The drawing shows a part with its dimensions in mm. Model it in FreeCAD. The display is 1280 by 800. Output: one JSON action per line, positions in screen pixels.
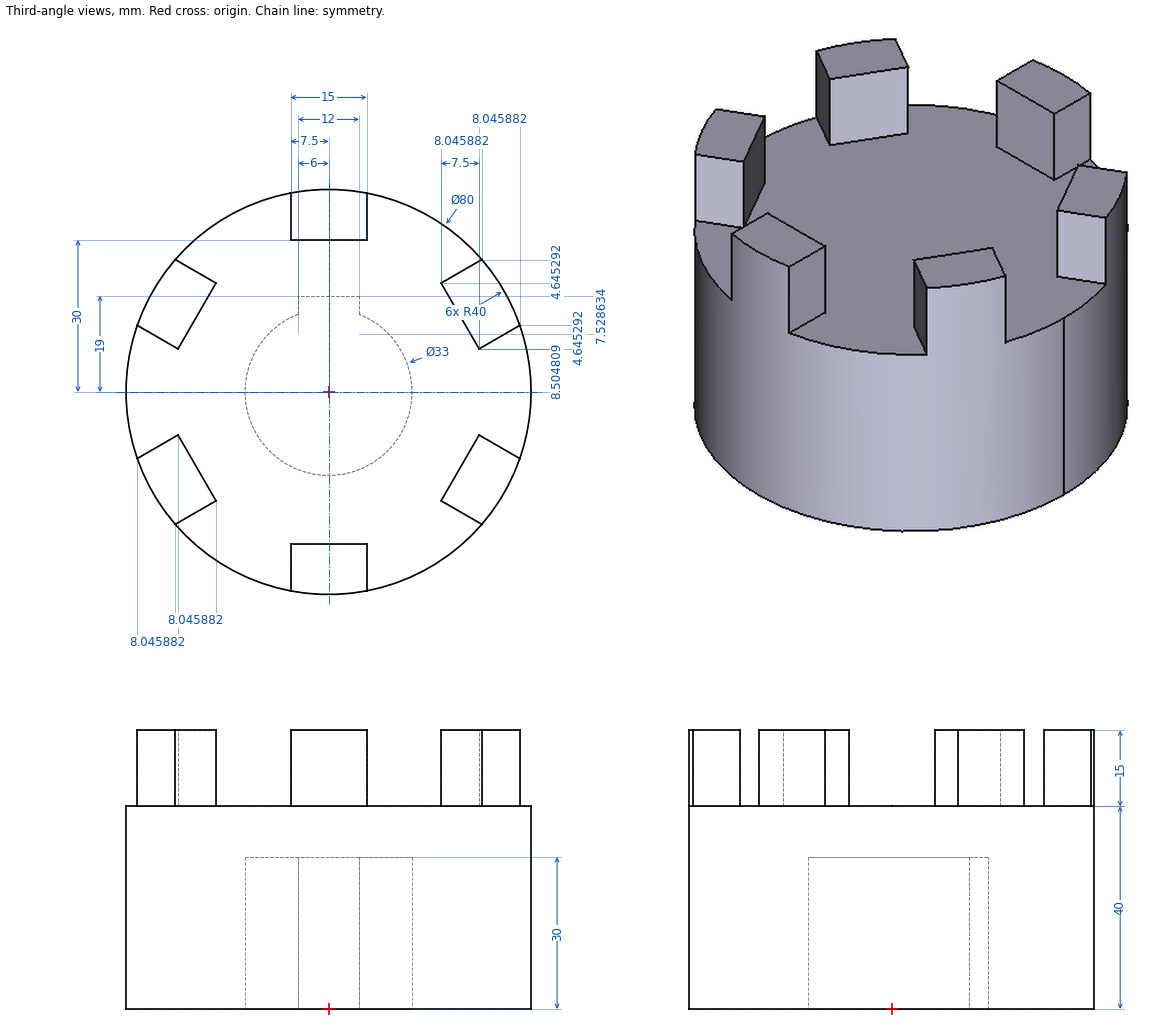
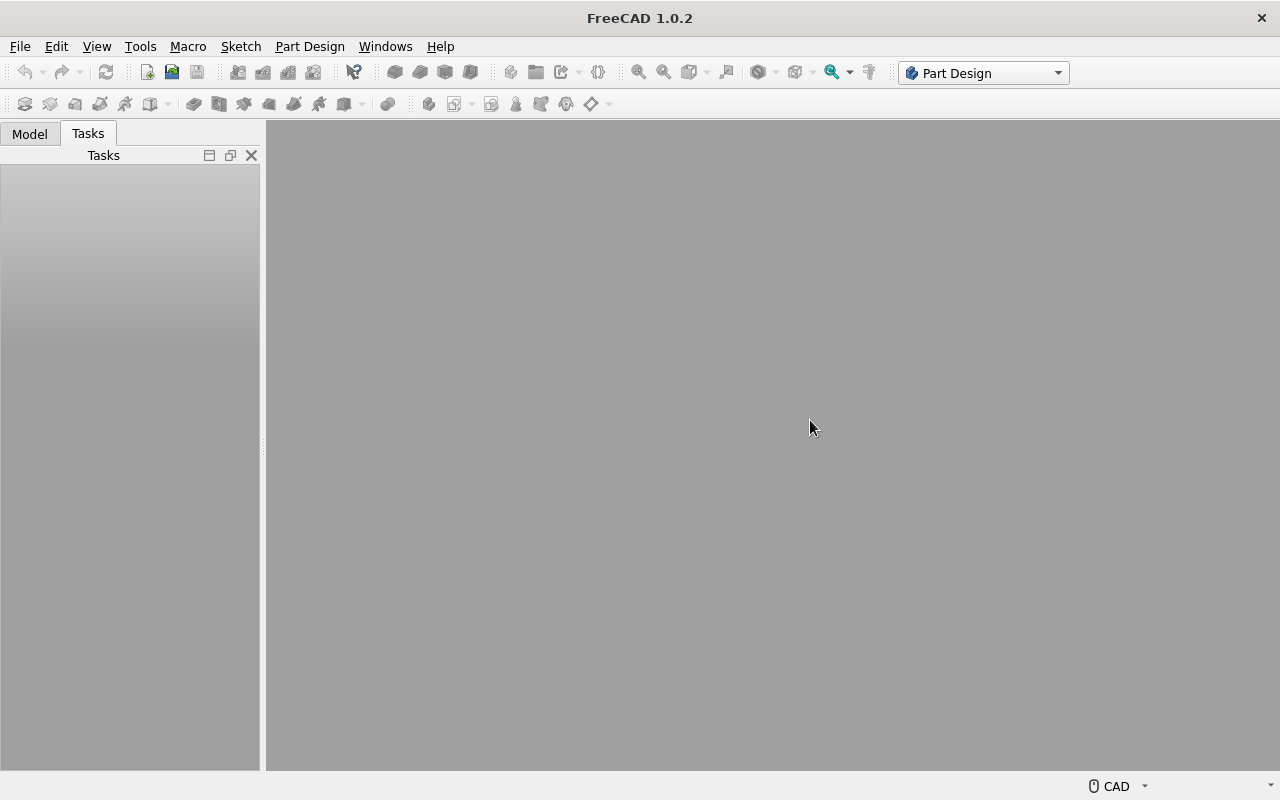
{"action": "key", "text": "ctrl+n"}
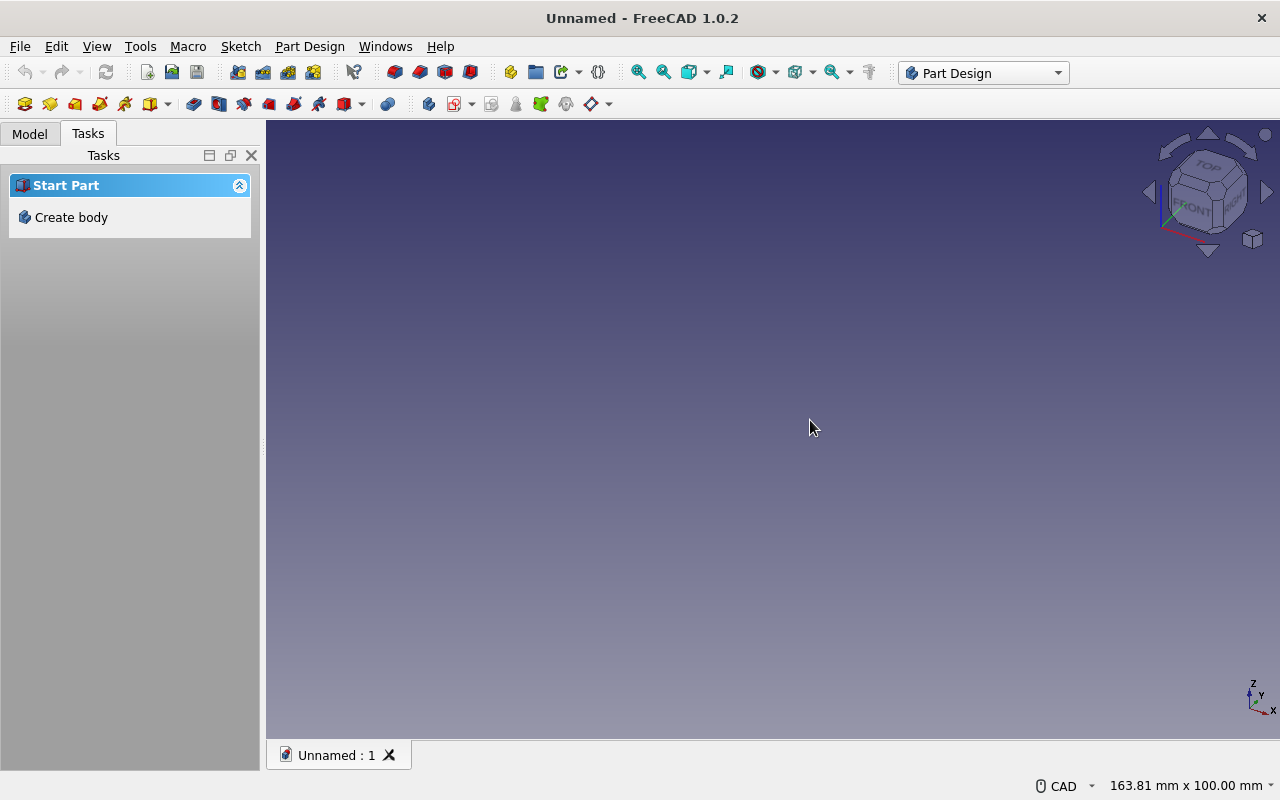
{"action": "left_click", "coordinate": [454, 104]}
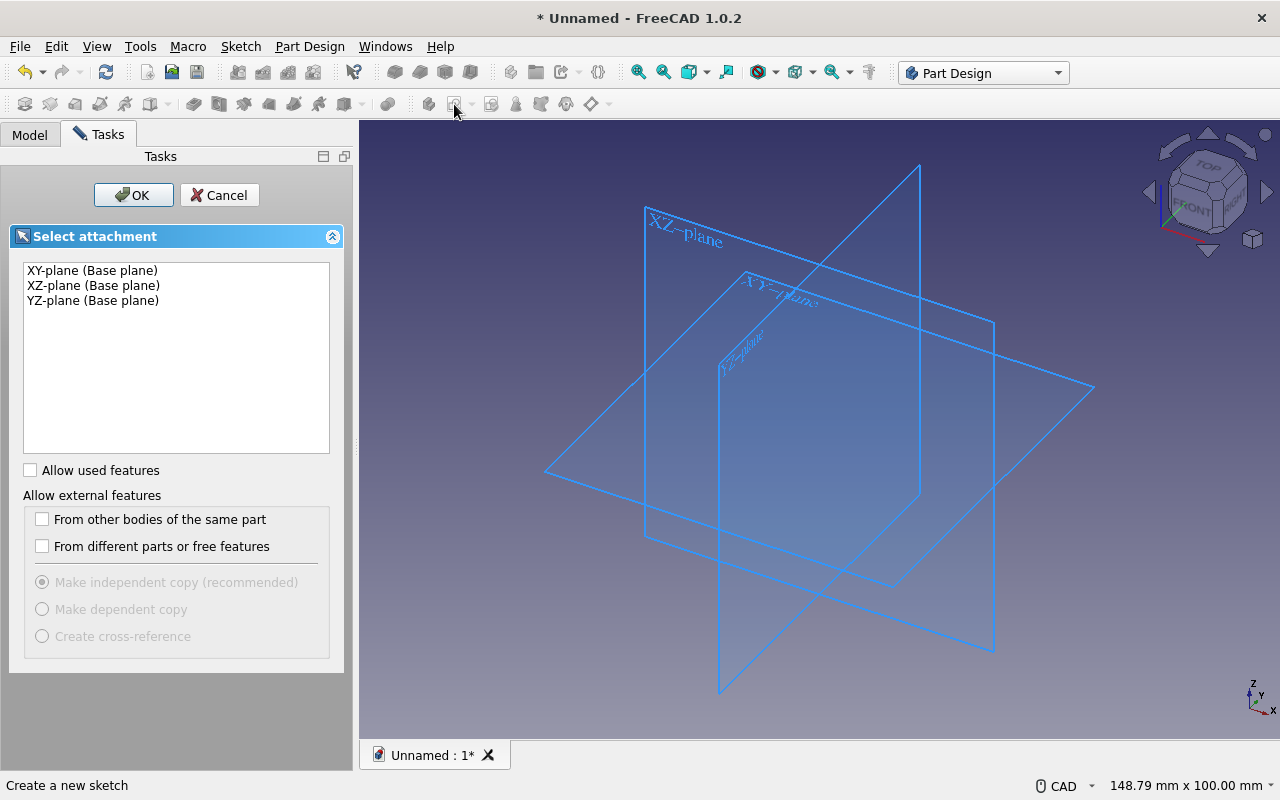
{"action": "left_click", "coordinate": [84, 270]}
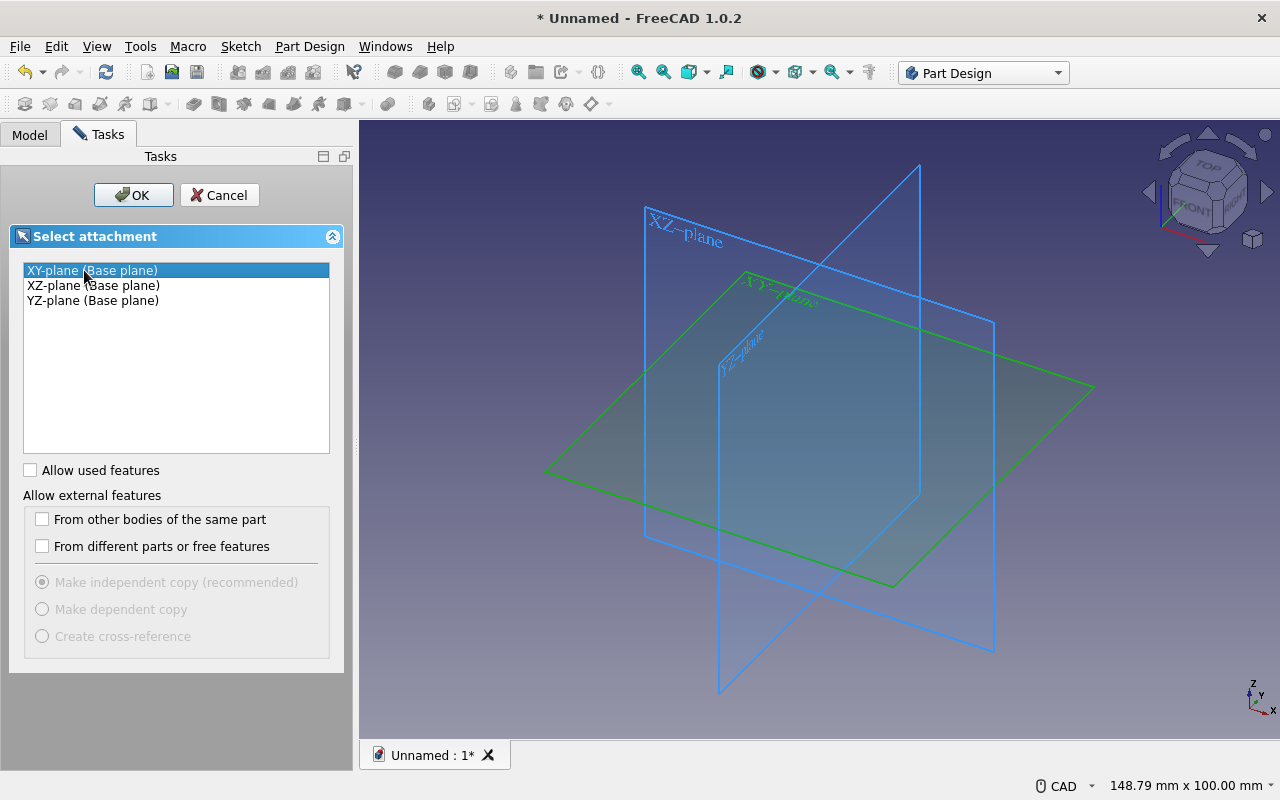
{"action": "left_click", "coordinate": [134, 195]}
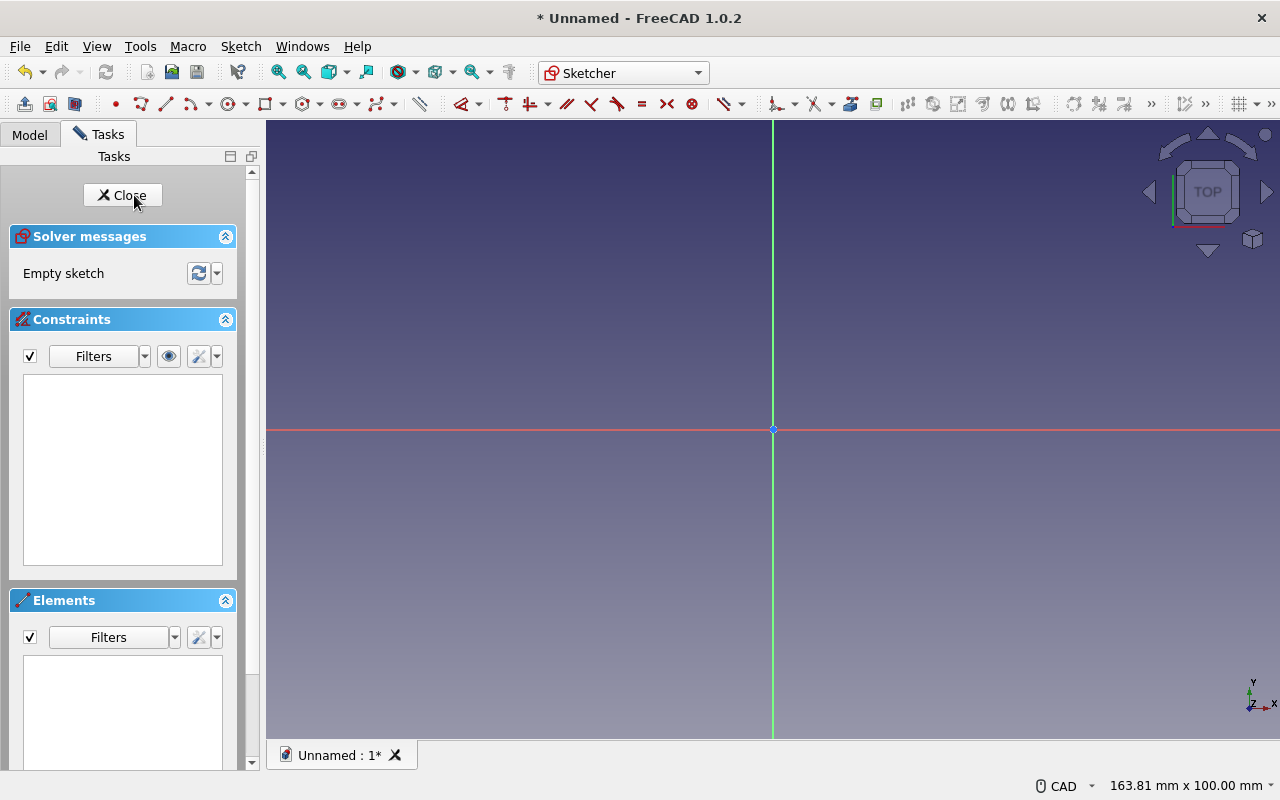
{"action": "key", "text": "g c"}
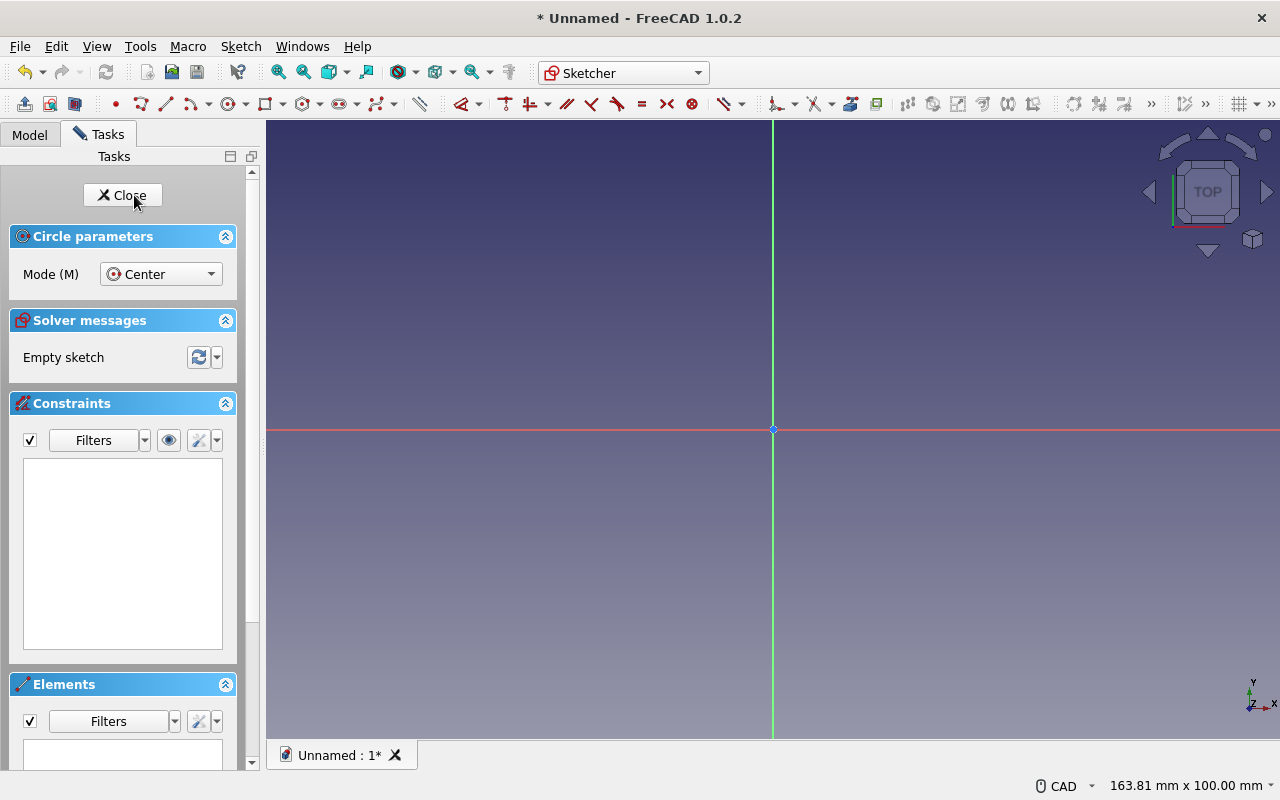
{"action": "left_click", "coordinate": [773, 430]}
{"action": "mouse_move", "coordinate": [948, 254]}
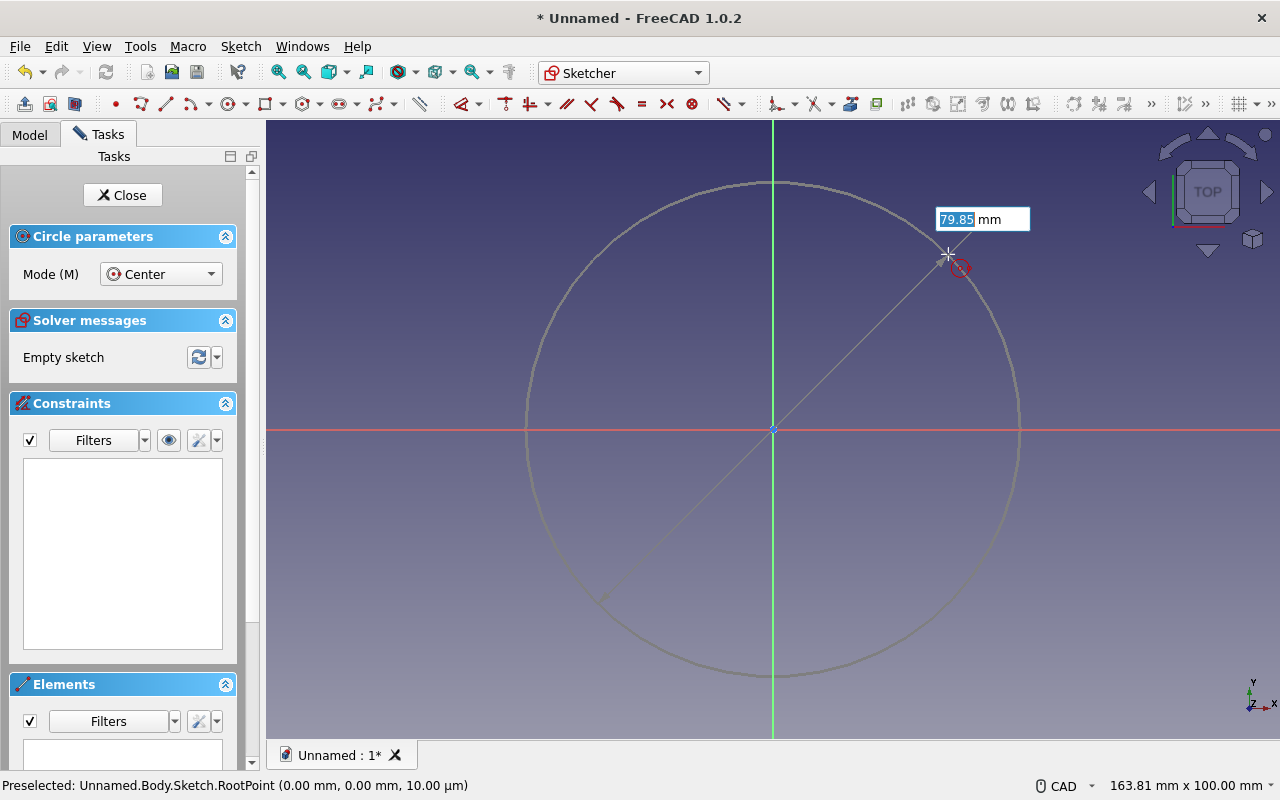
{"action": "type", "text": "80"}
{"action": "key", "text": "Return"}
{"action": "key", "text": "Escape"}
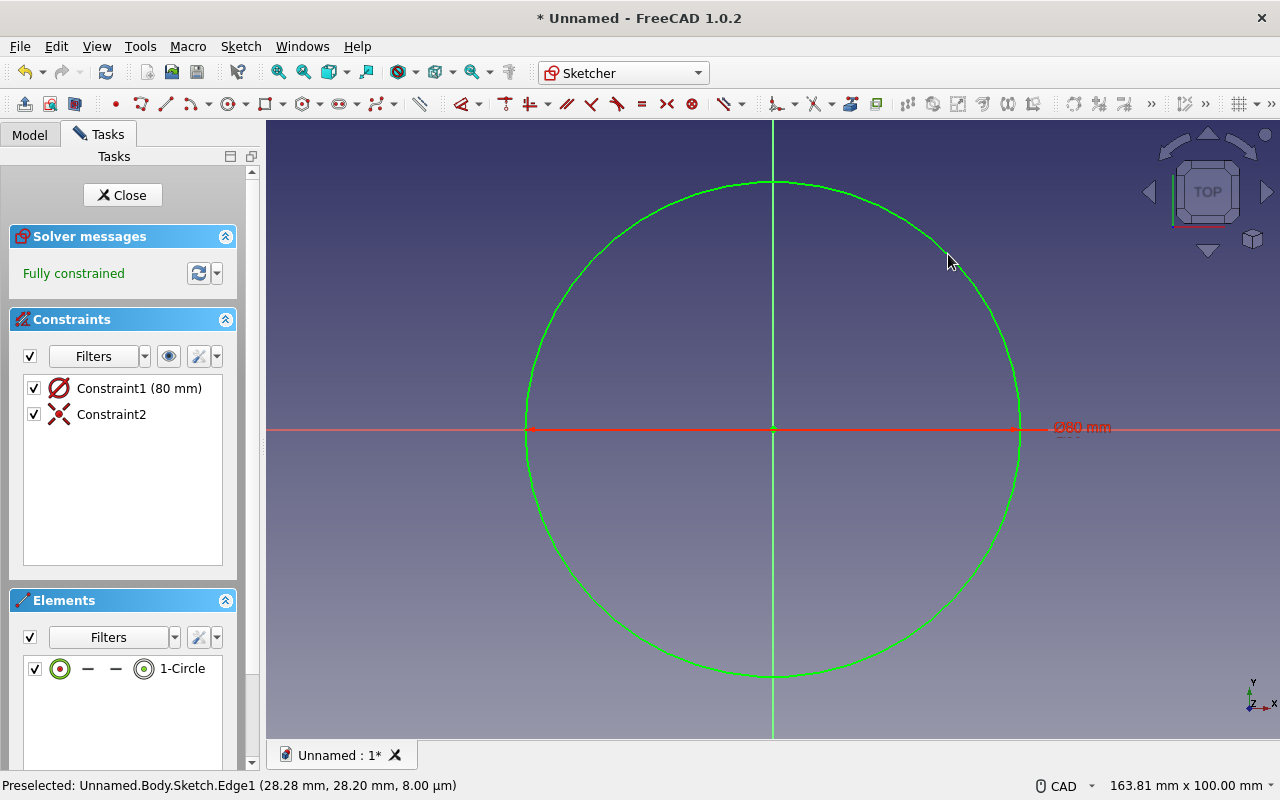
{"action": "left_click", "coordinate": [123, 195]}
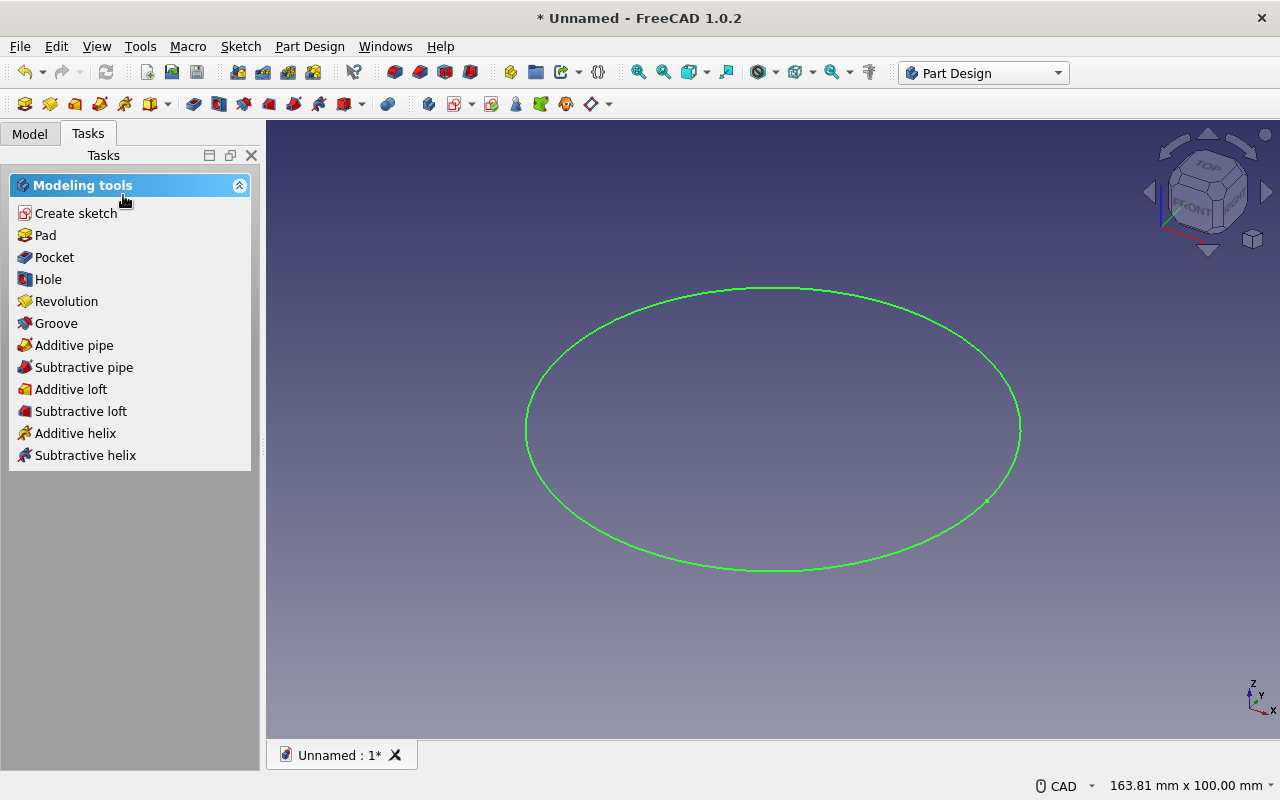
{"action": "left_click", "coordinate": [25, 104]}